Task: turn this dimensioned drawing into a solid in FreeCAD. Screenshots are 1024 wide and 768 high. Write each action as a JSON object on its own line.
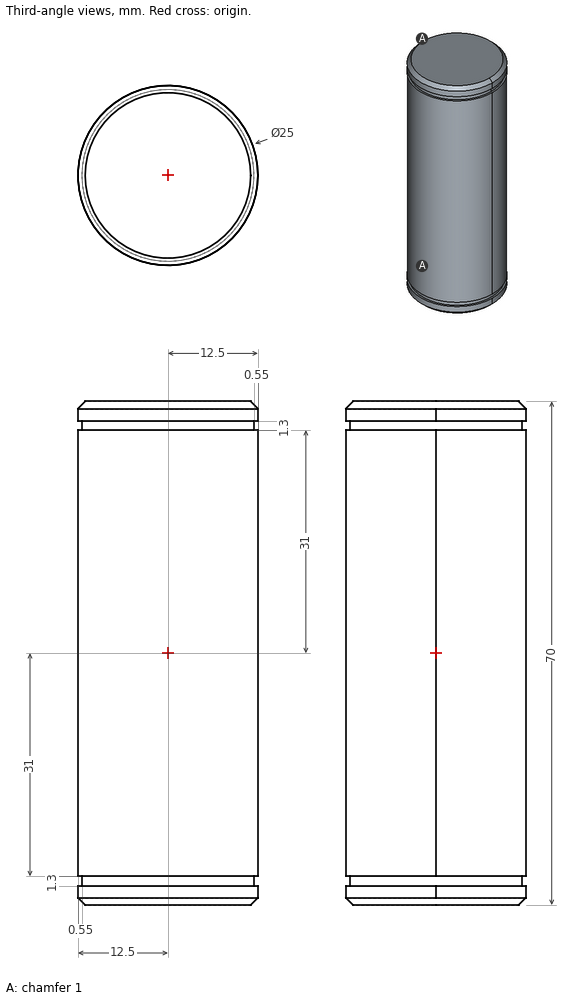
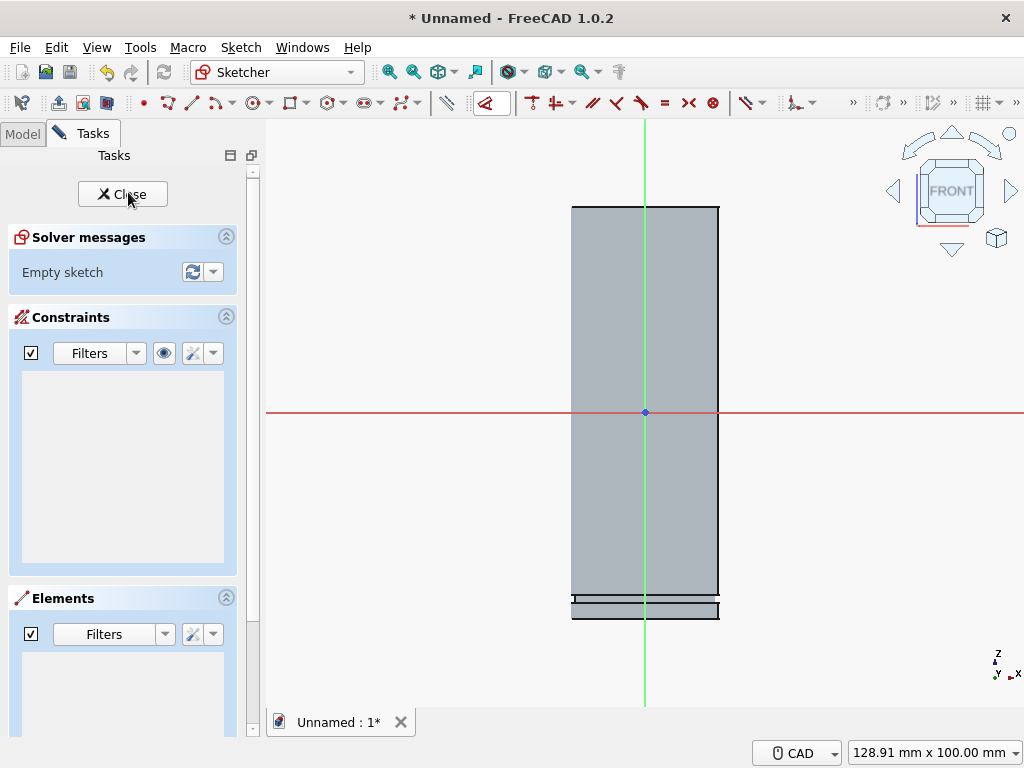
{"action": "scroll", "coordinate": [724, 217], "scroll_direction": "up", "scroll_amount": 15}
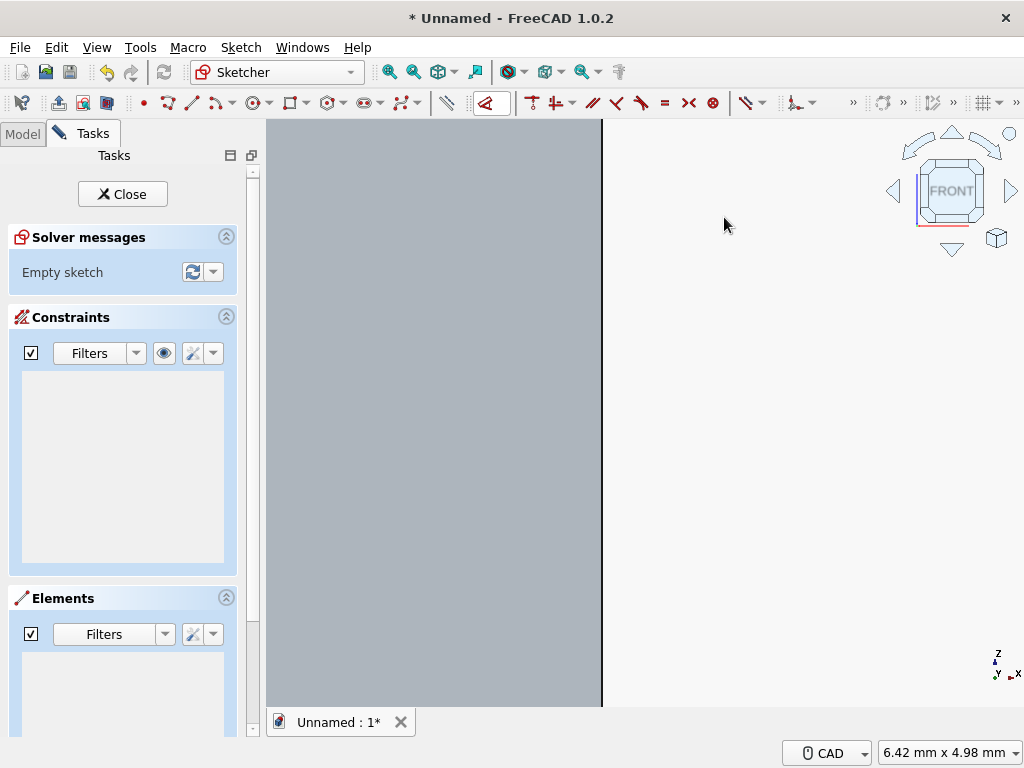
{"action": "scroll", "coordinate": [564, 412], "scroll_direction": "up", "scroll_amount": 4}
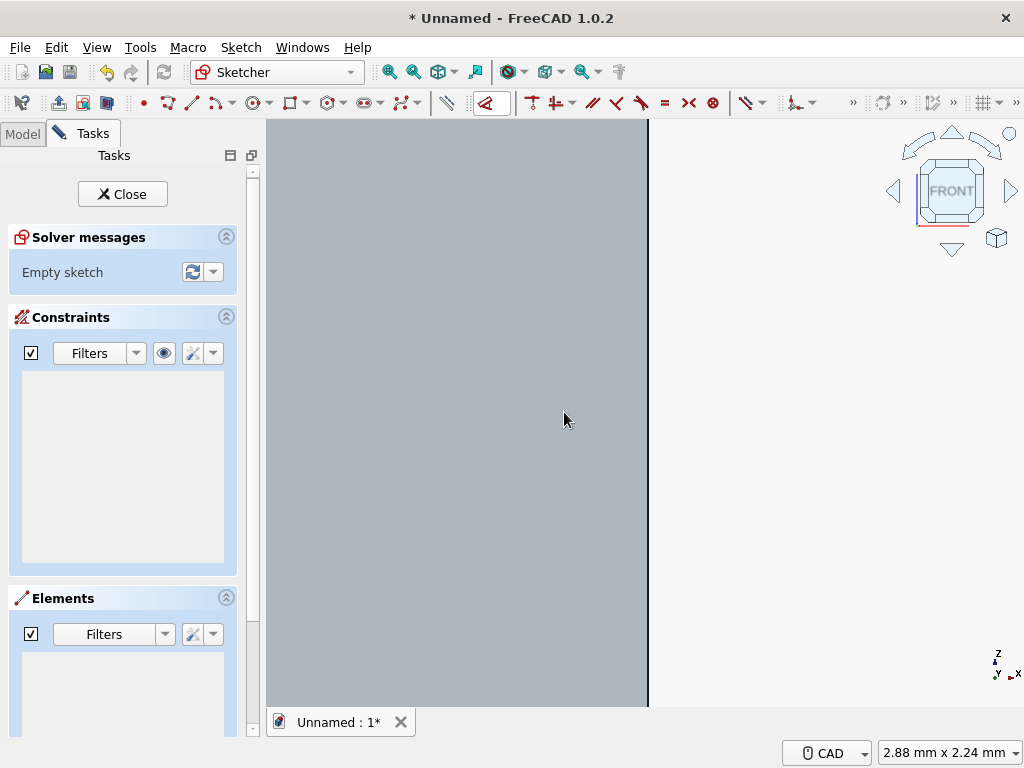
{"action": "key", "text": "g r"}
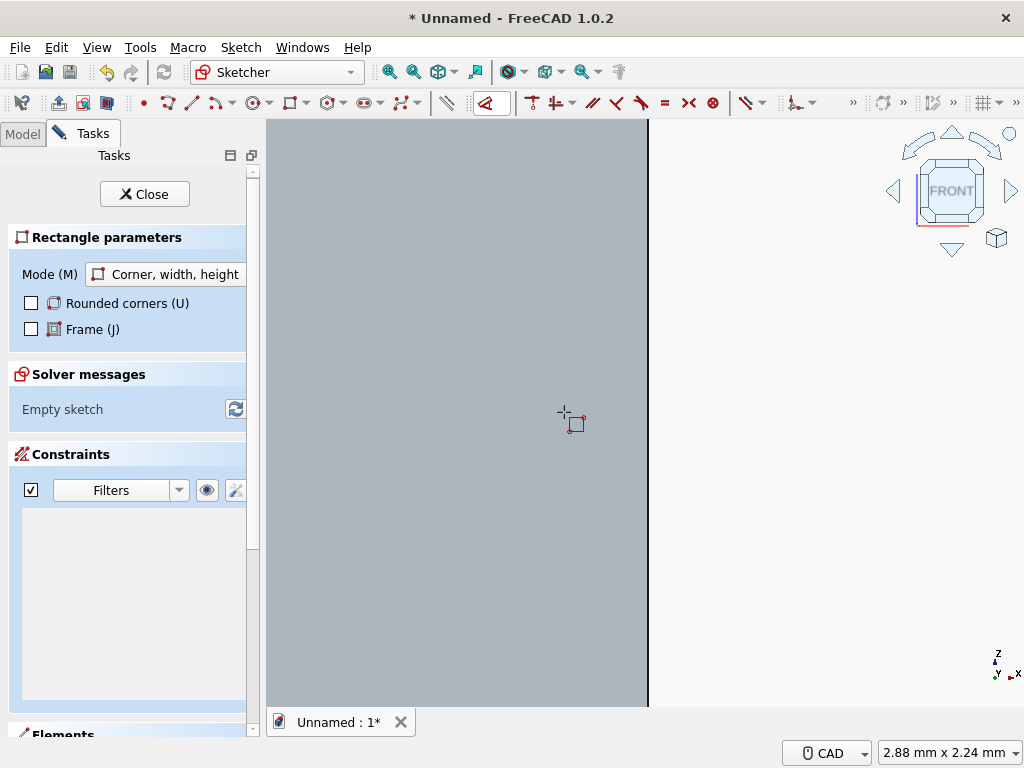
{"action": "left_click", "coordinate": [503, 242]}
{"action": "left_click", "coordinate": [648, 584]}
{"action": "key", "text": "Escape"}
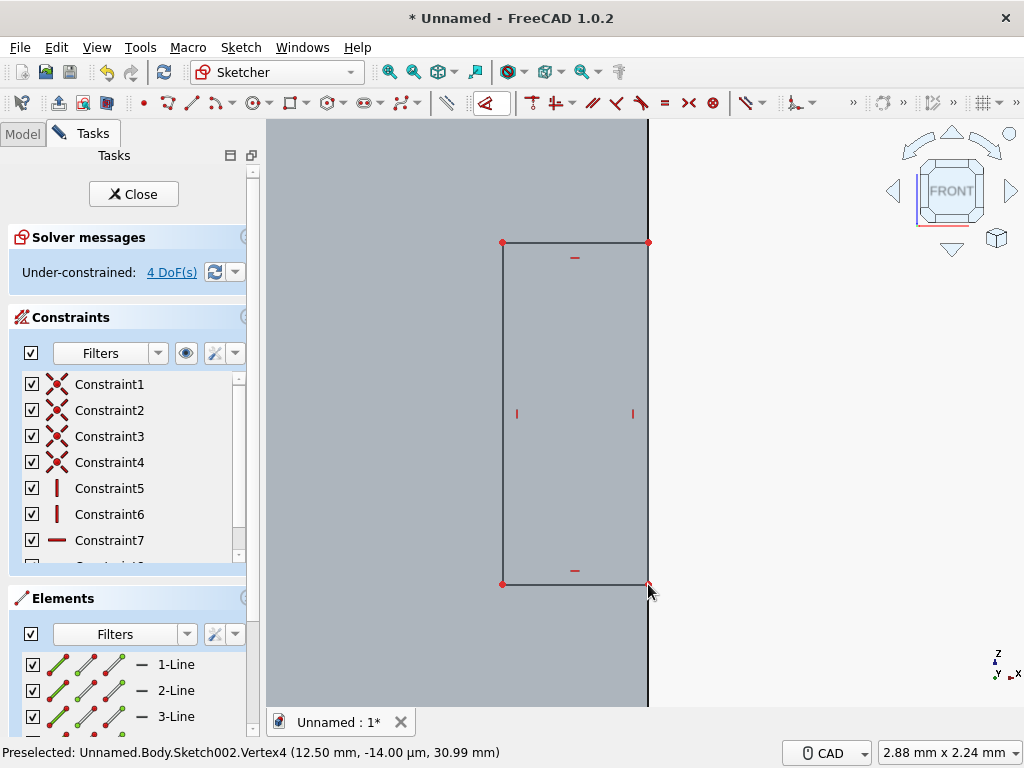
{"action": "key", "text": "d"}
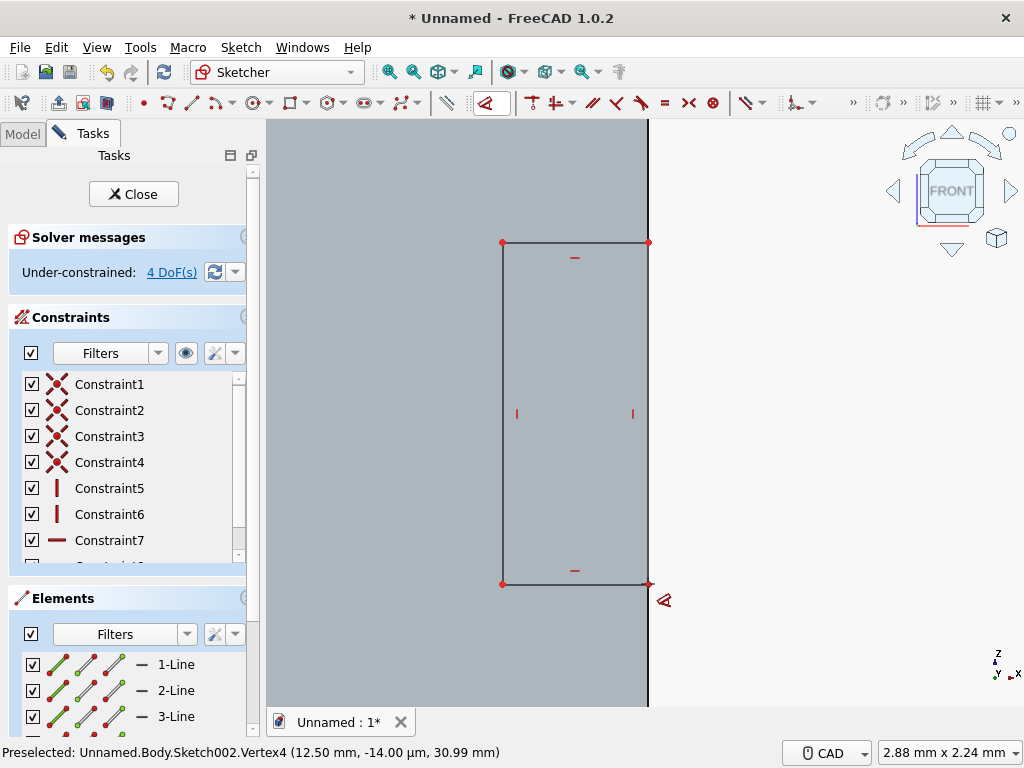
{"action": "left_click", "coordinate": [503, 346]}
{"action": "left_click", "coordinate": [469, 414]}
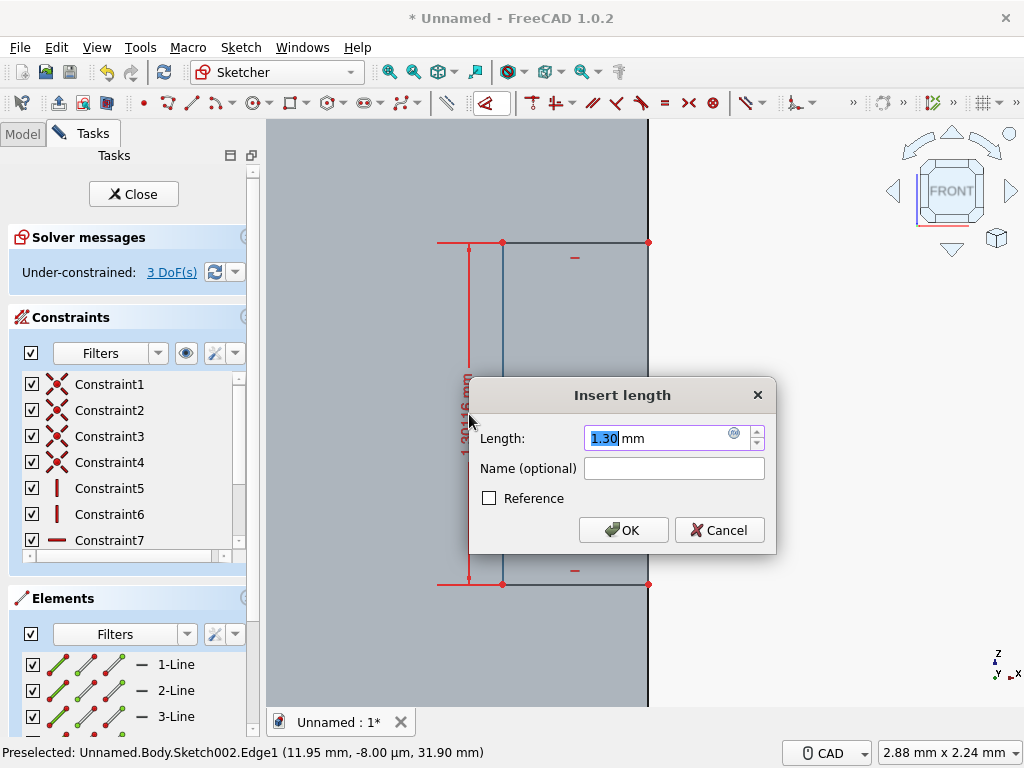
{"action": "type", "text": "1.3"}
{"action": "key", "text": "Return"}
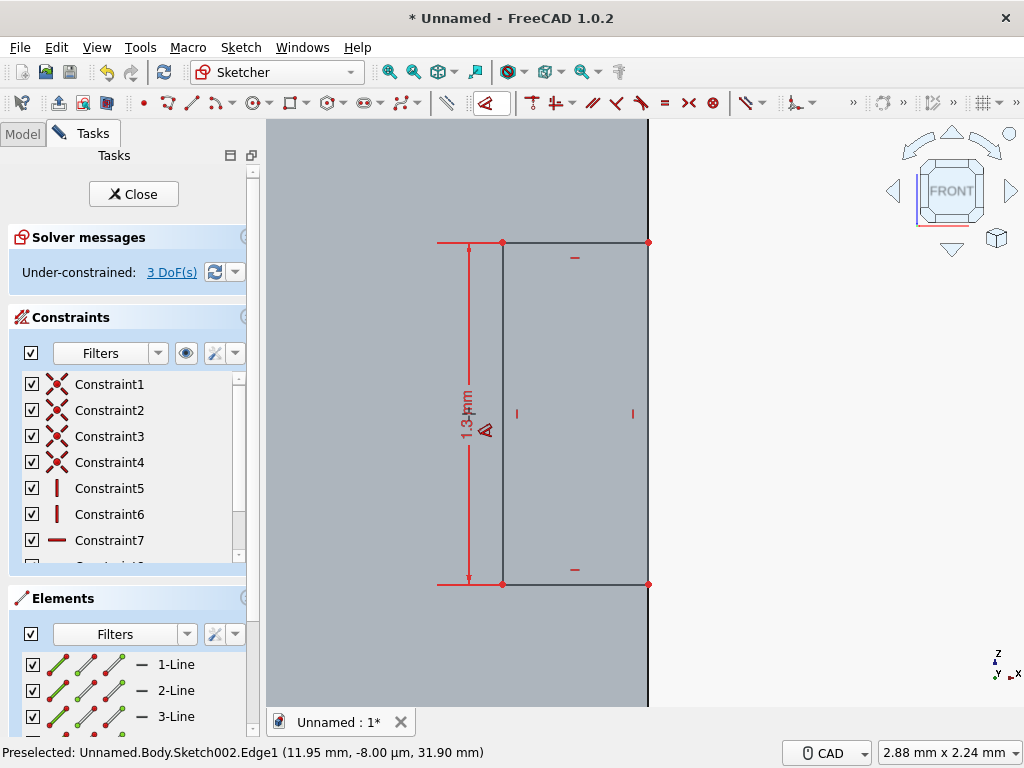
{"action": "left_click", "coordinate": [503, 585]}
{"action": "left_click", "coordinate": [537, 632]}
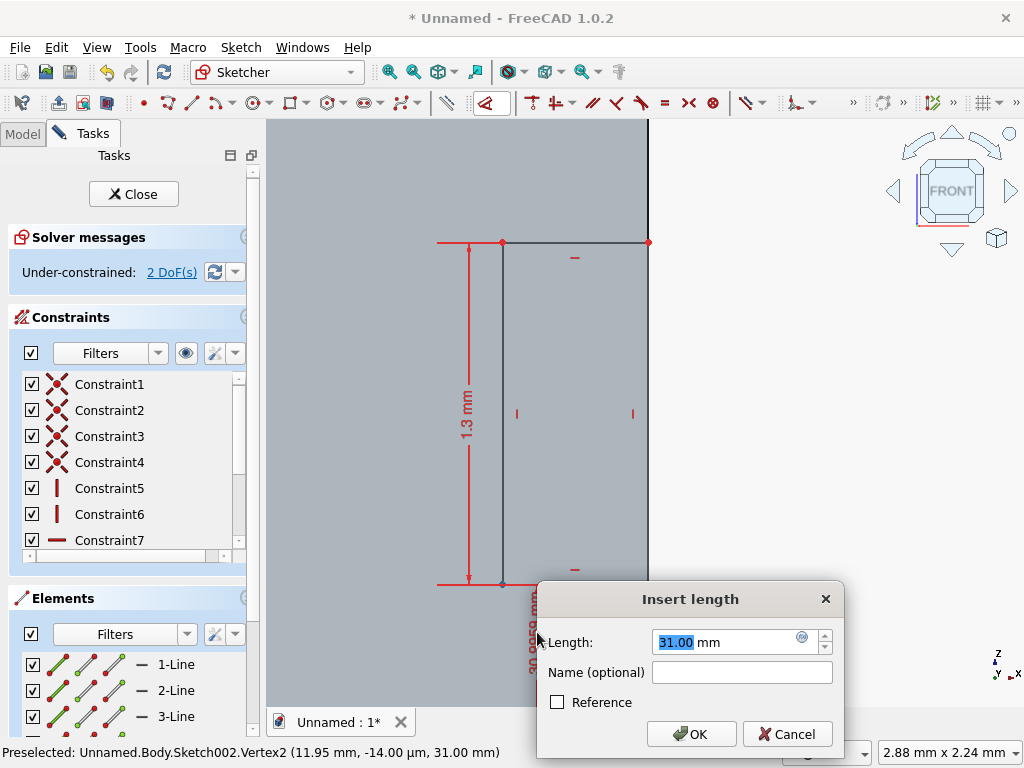
{"action": "type", "text": "31"}
{"action": "key", "text": "Return"}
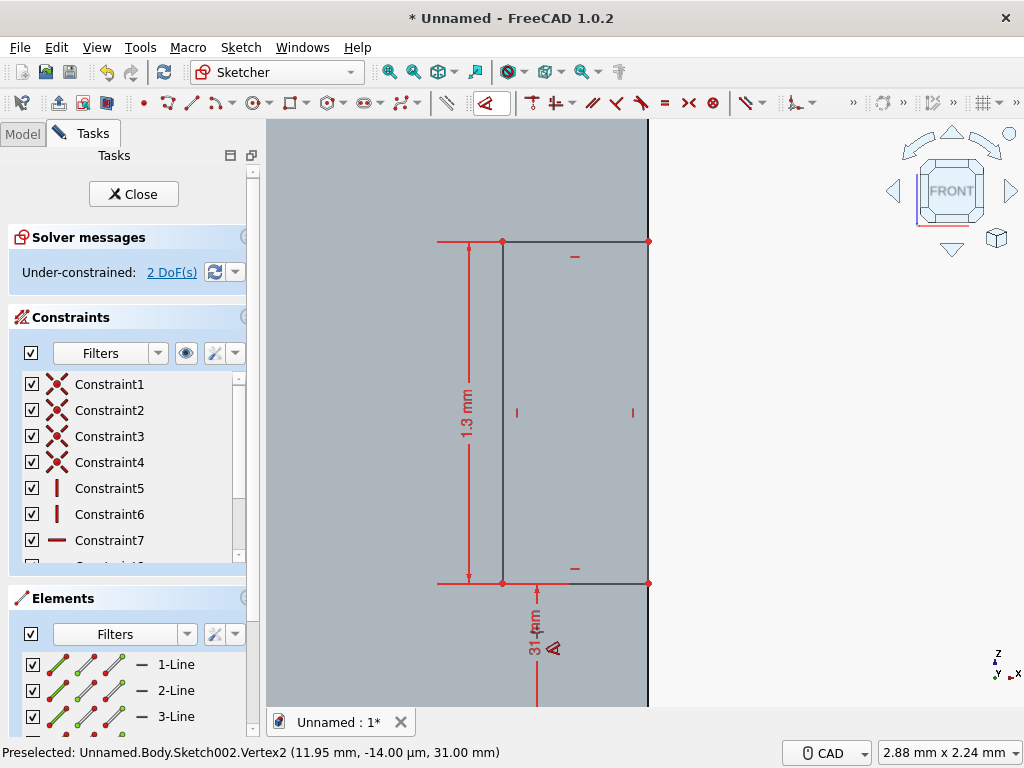
{"action": "left_click", "coordinate": [546, 584]}
{"action": "left_click", "coordinate": [609, 618]}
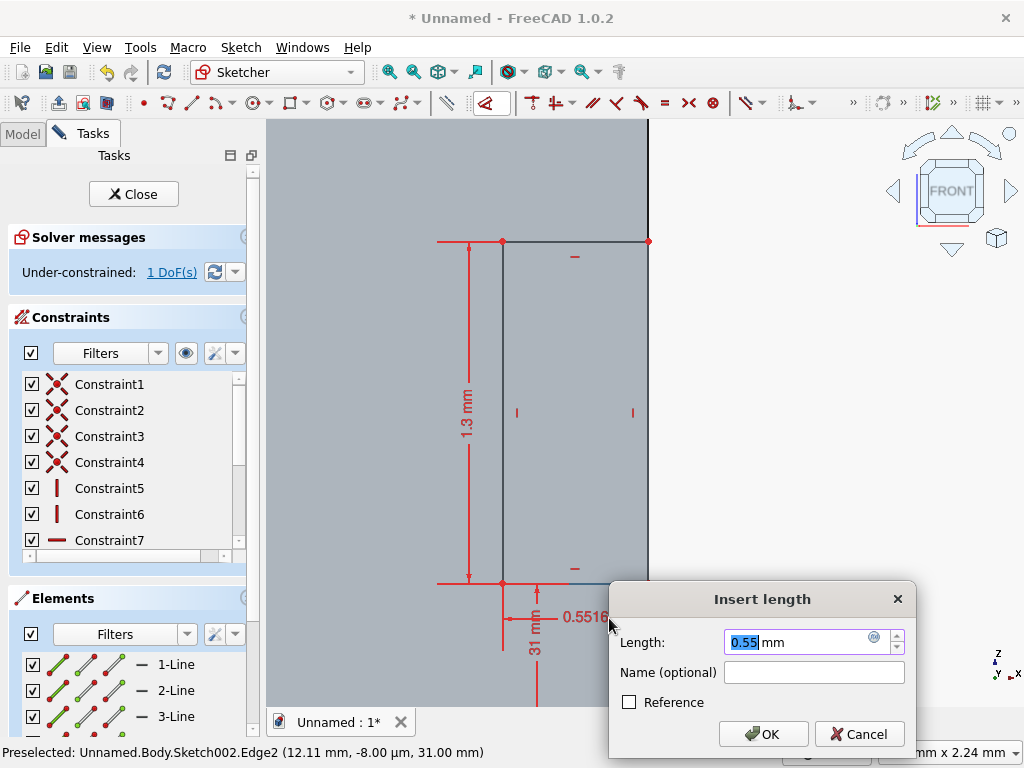
{"action": "type", "text": "0.55"}
{"action": "key", "text": "Return"}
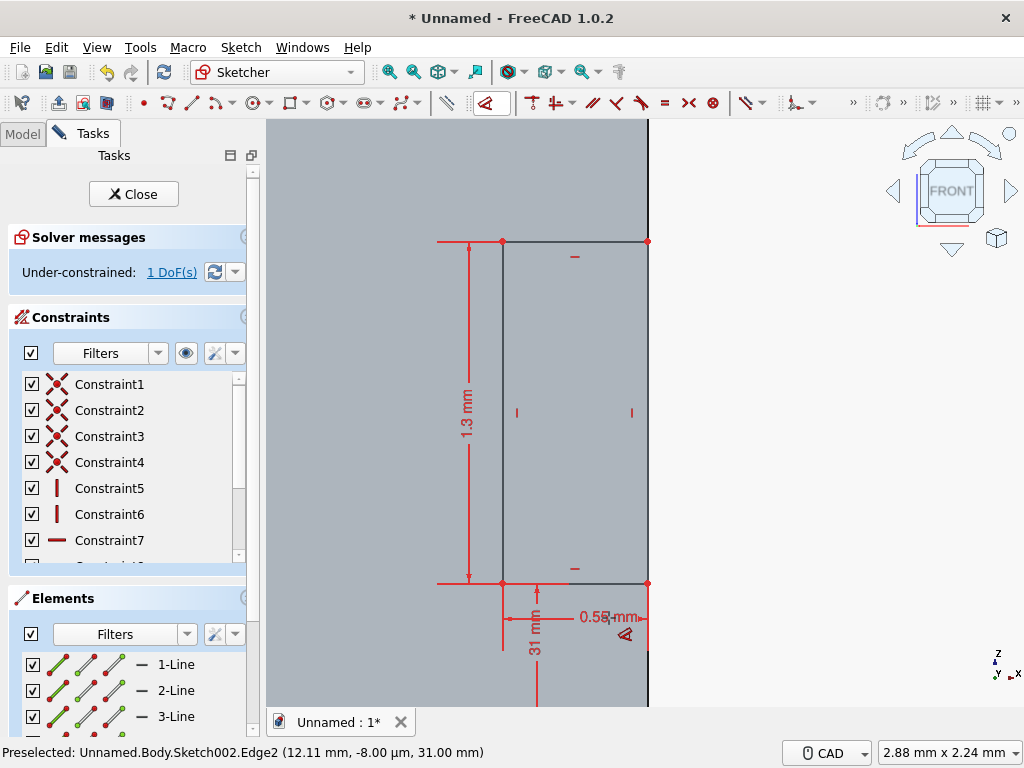
{"action": "left_click", "coordinate": [648, 584]}
{"action": "left_click", "coordinate": [471, 550]}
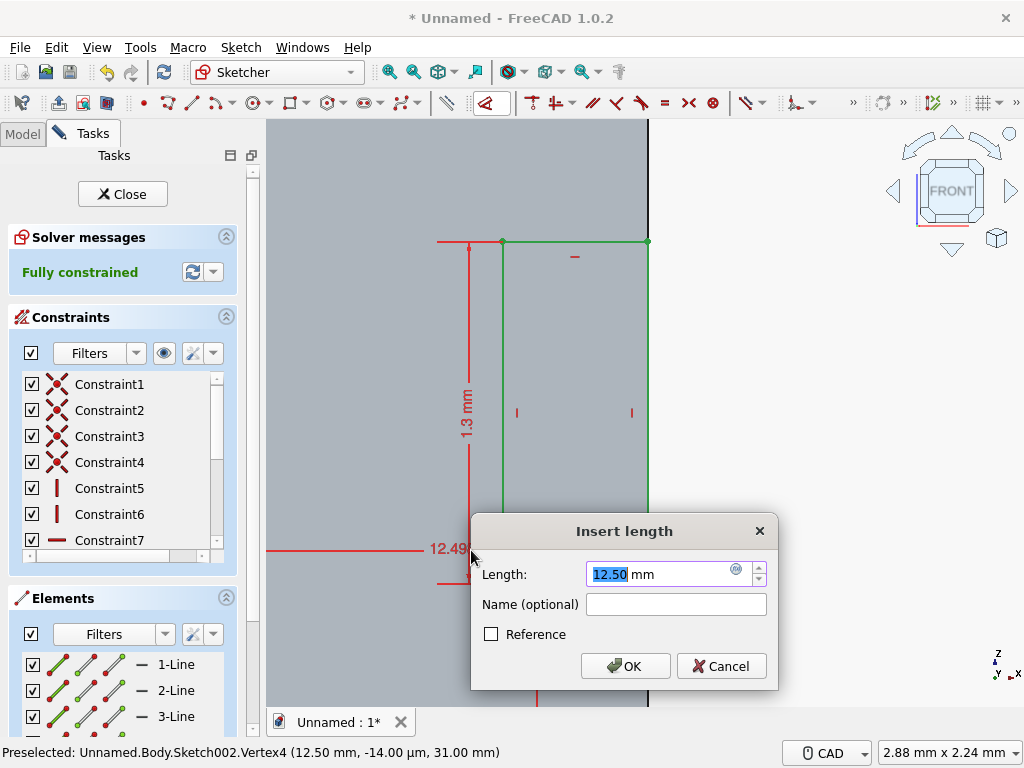
{"action": "type", "text": "12.5"}
{"action": "key", "text": "Return"}
{"action": "key", "text": "Escape"}